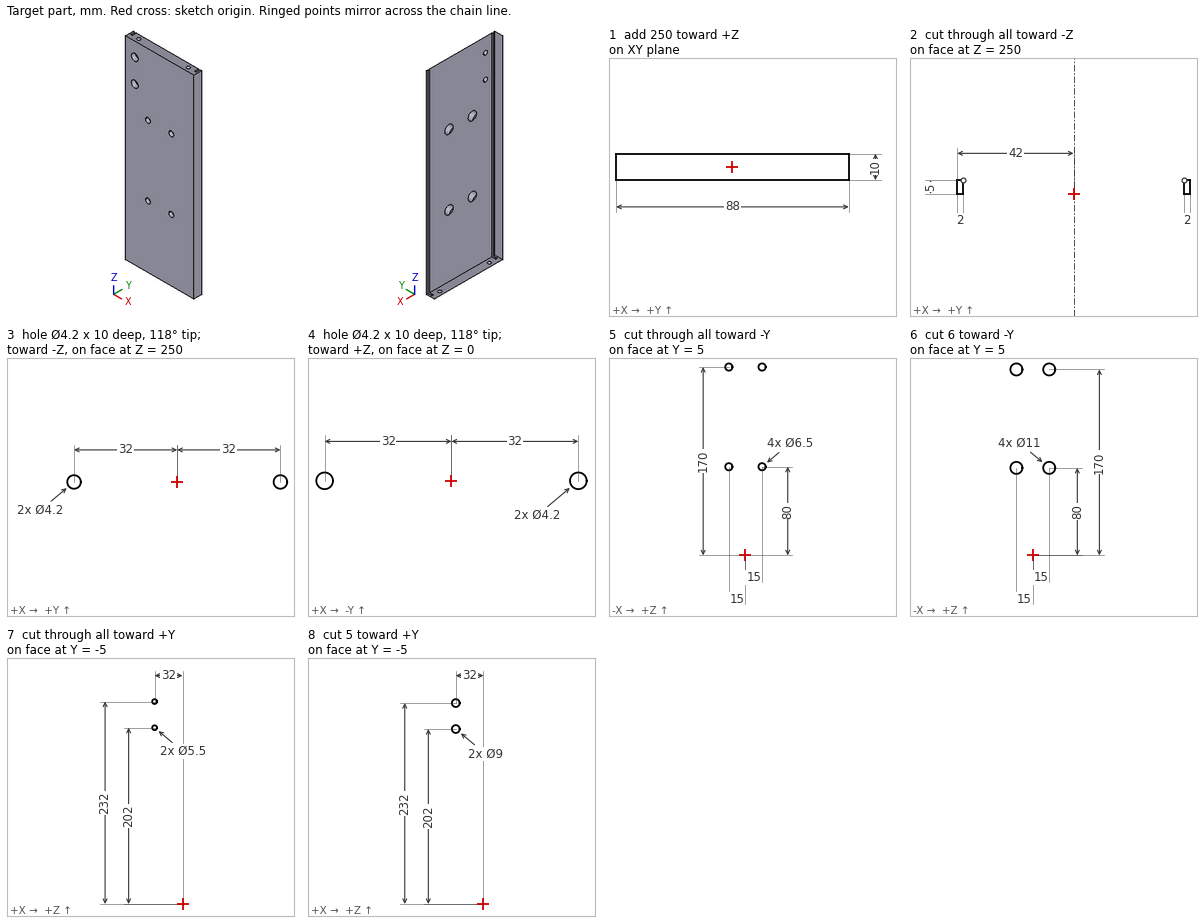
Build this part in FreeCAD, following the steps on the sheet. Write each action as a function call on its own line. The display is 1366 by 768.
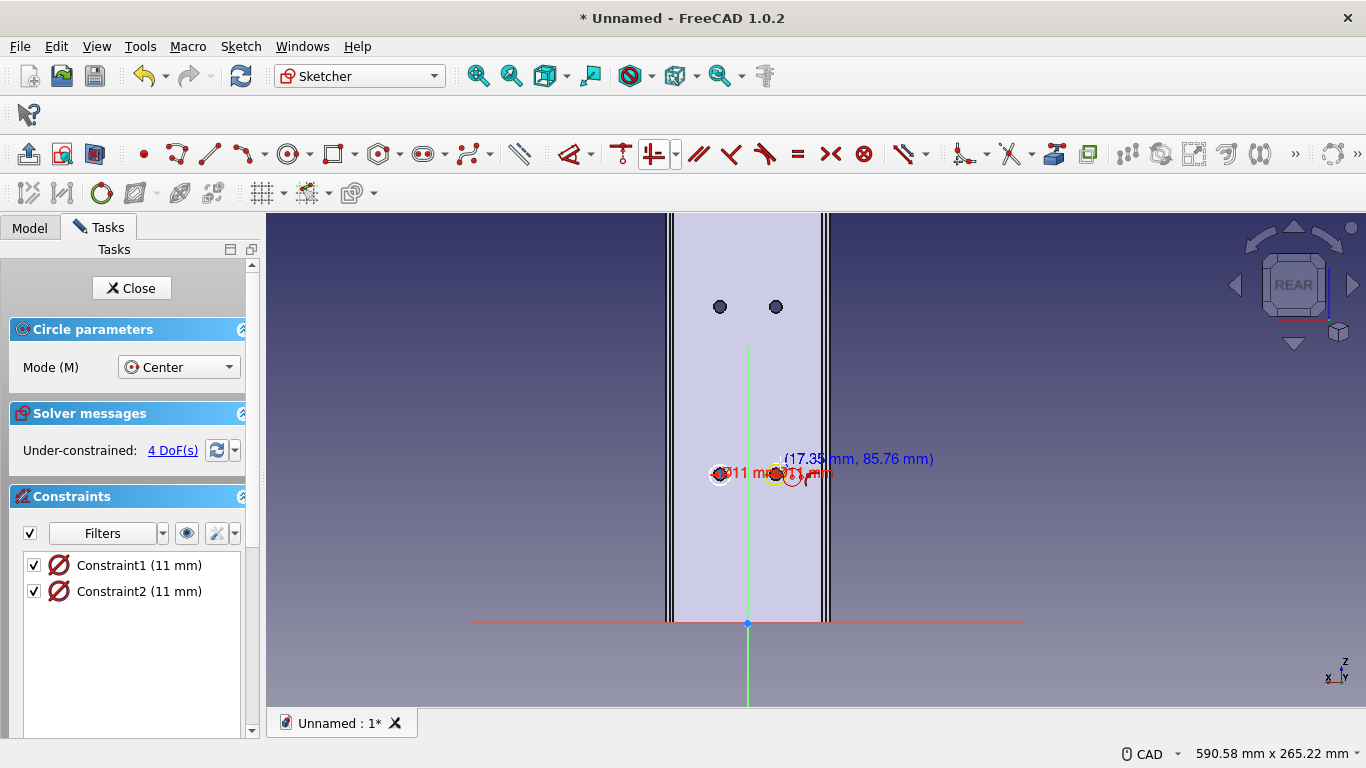
scroll(776, 307, up, 4)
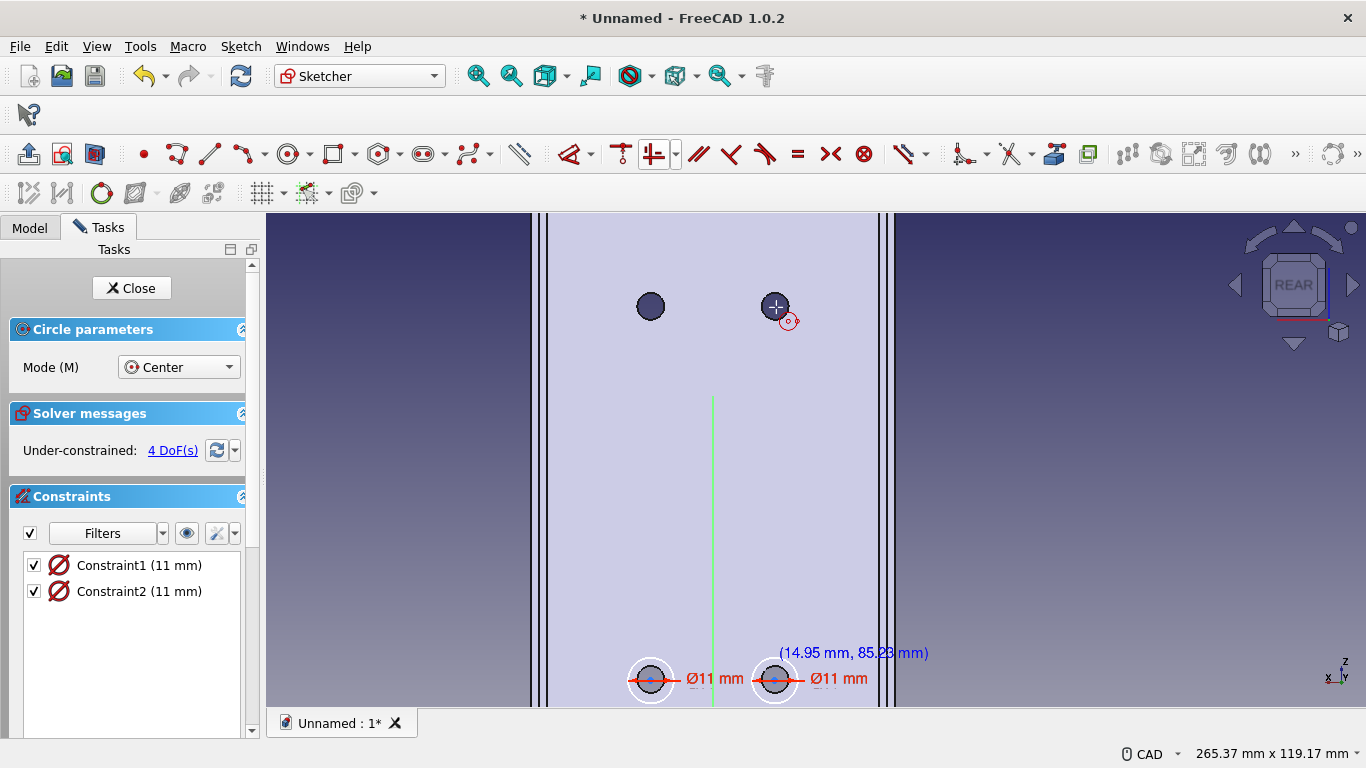
click(775, 306)
move(791, 290)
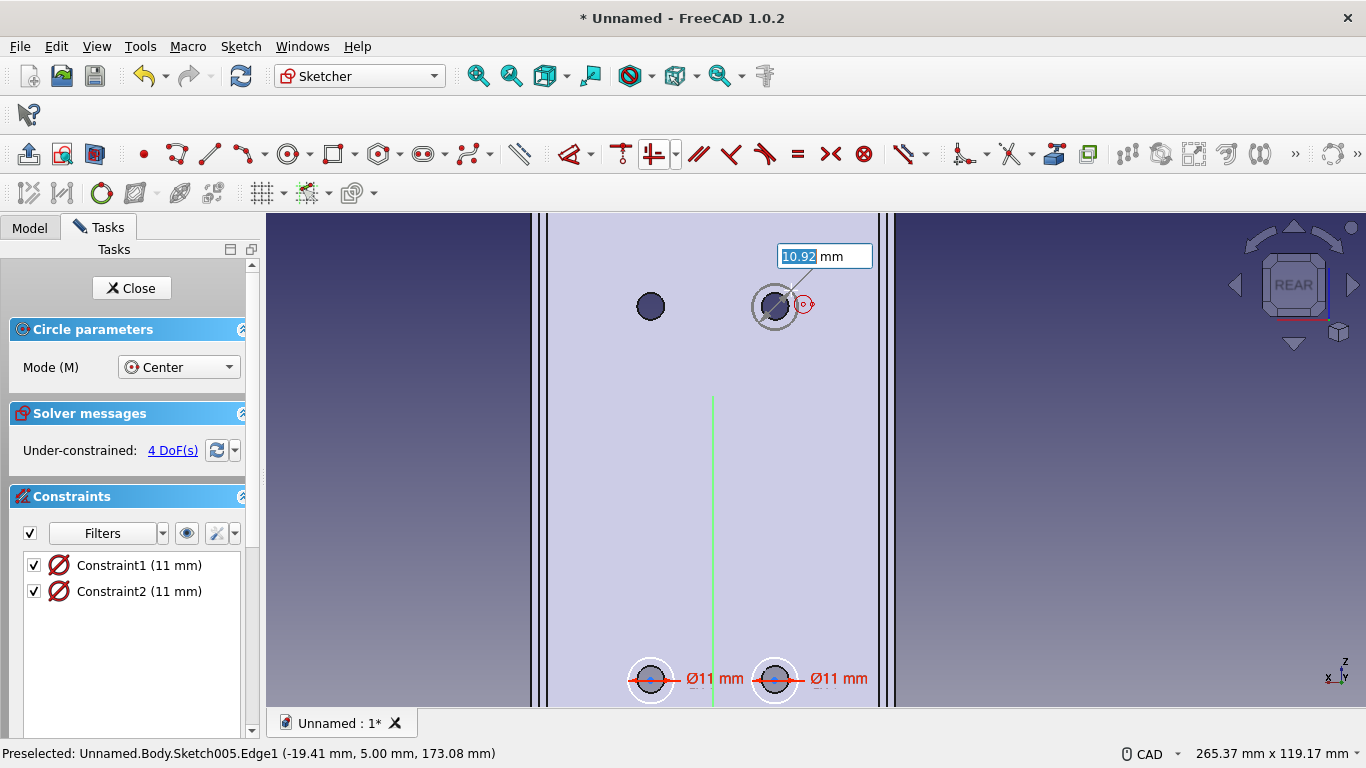
text(11)
key(Return)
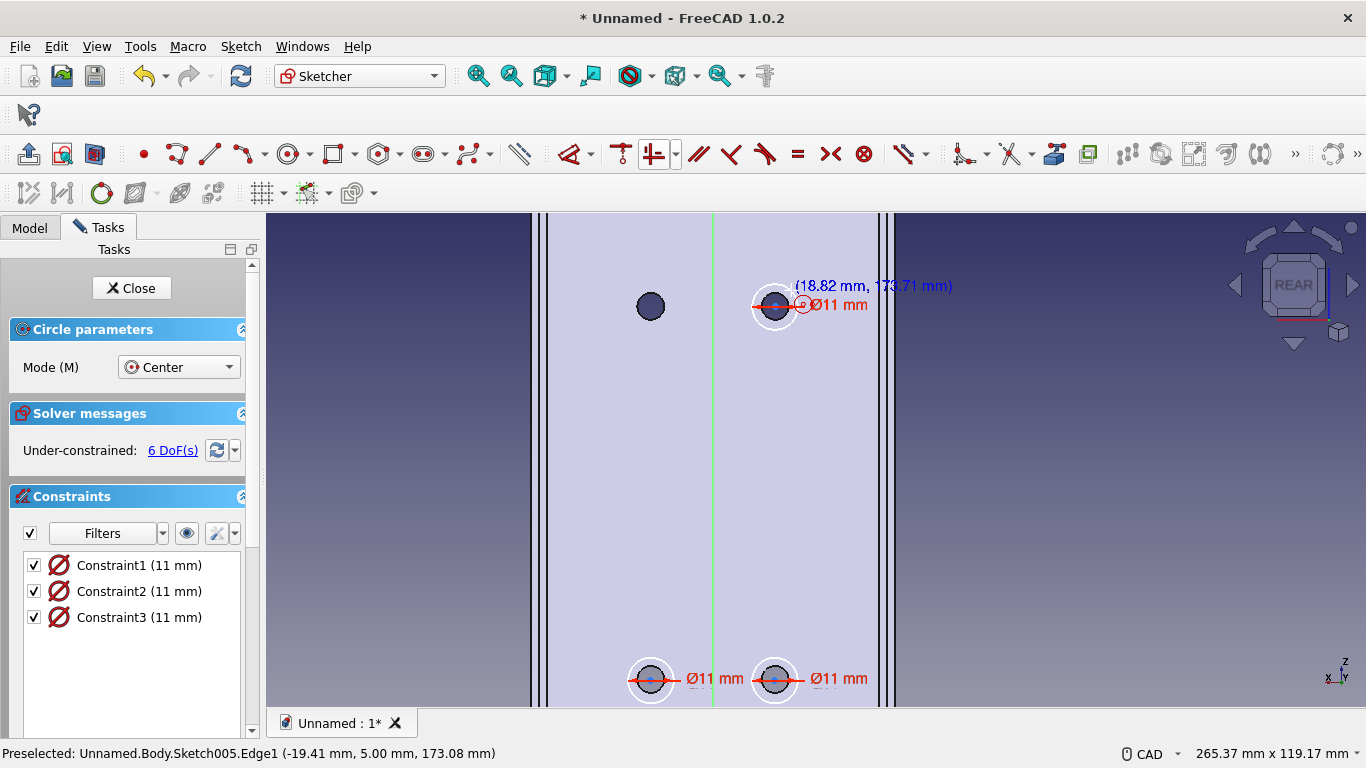
click(651, 306)
move(667, 290)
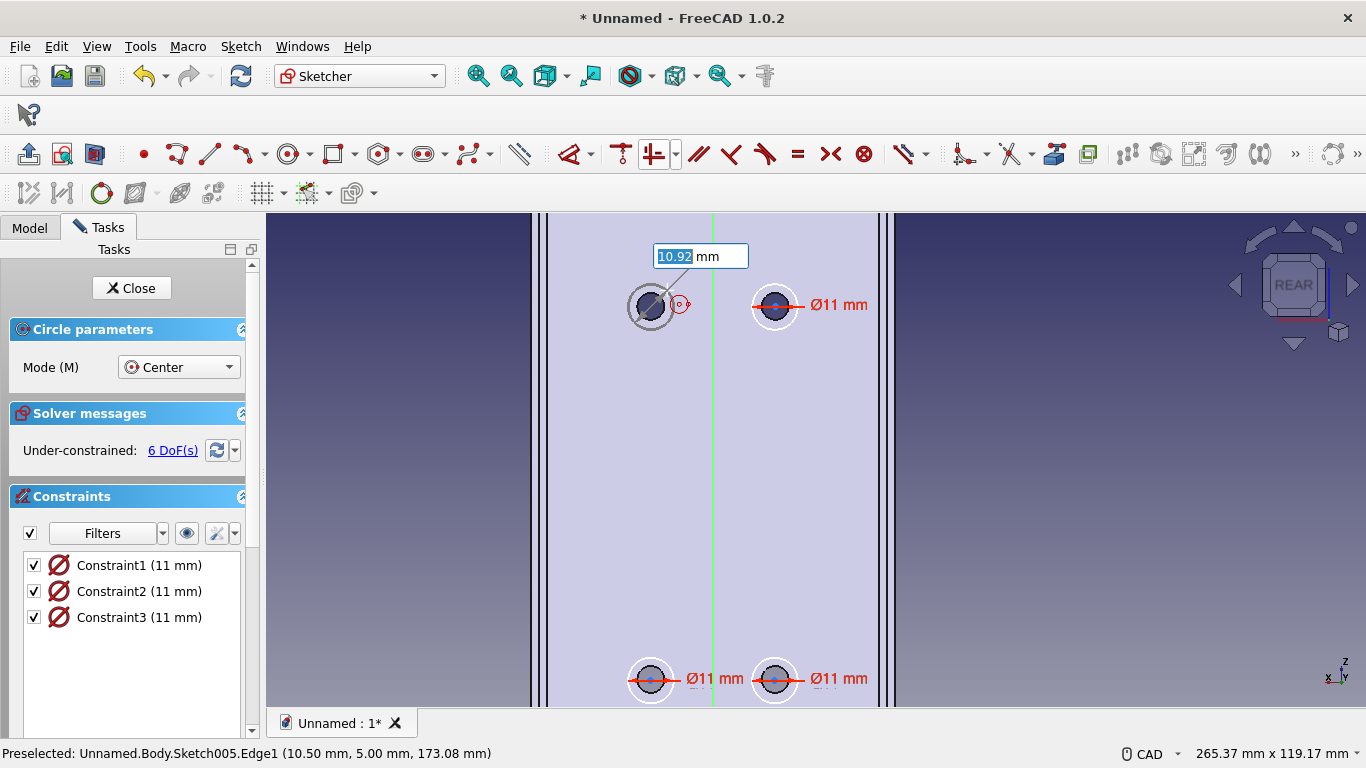
text(11)
key(Return)
key(Escape)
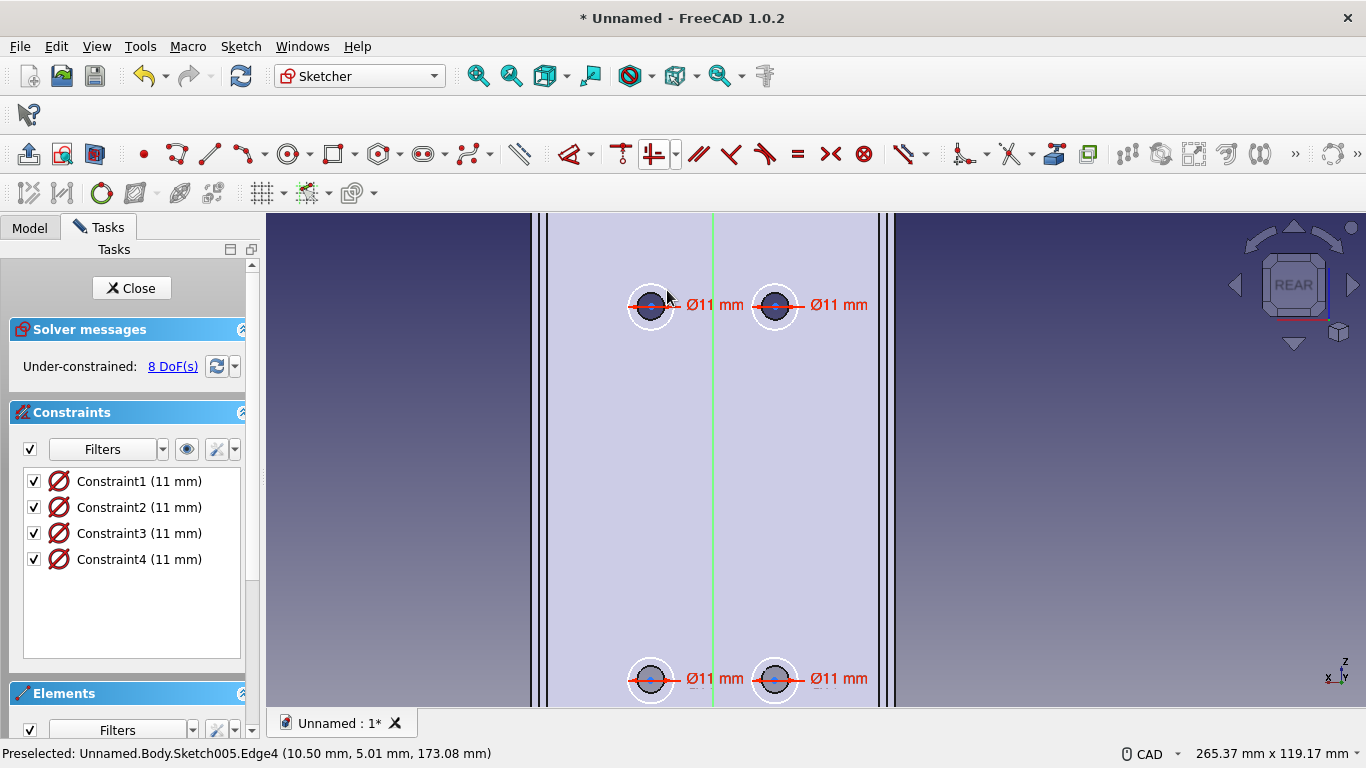
scroll(776, 307, down, 4)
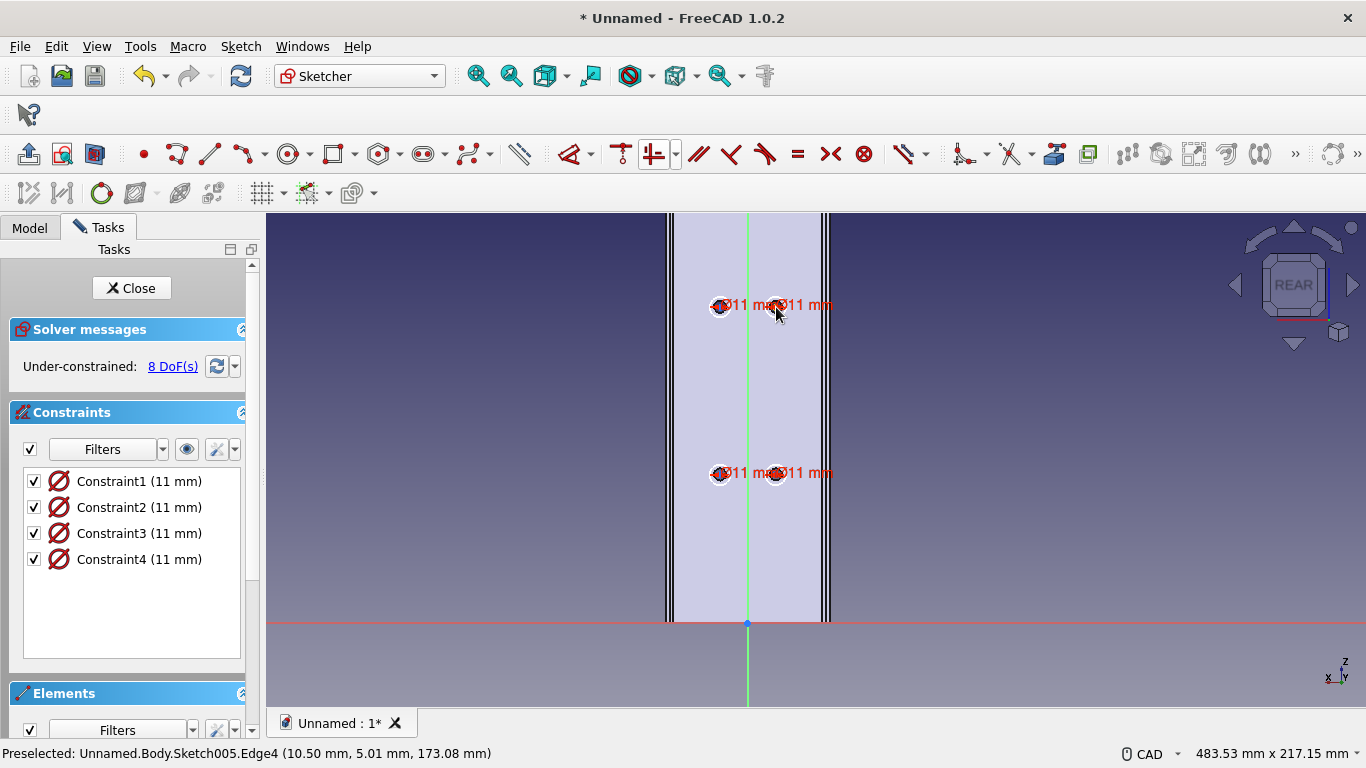
click(776, 475)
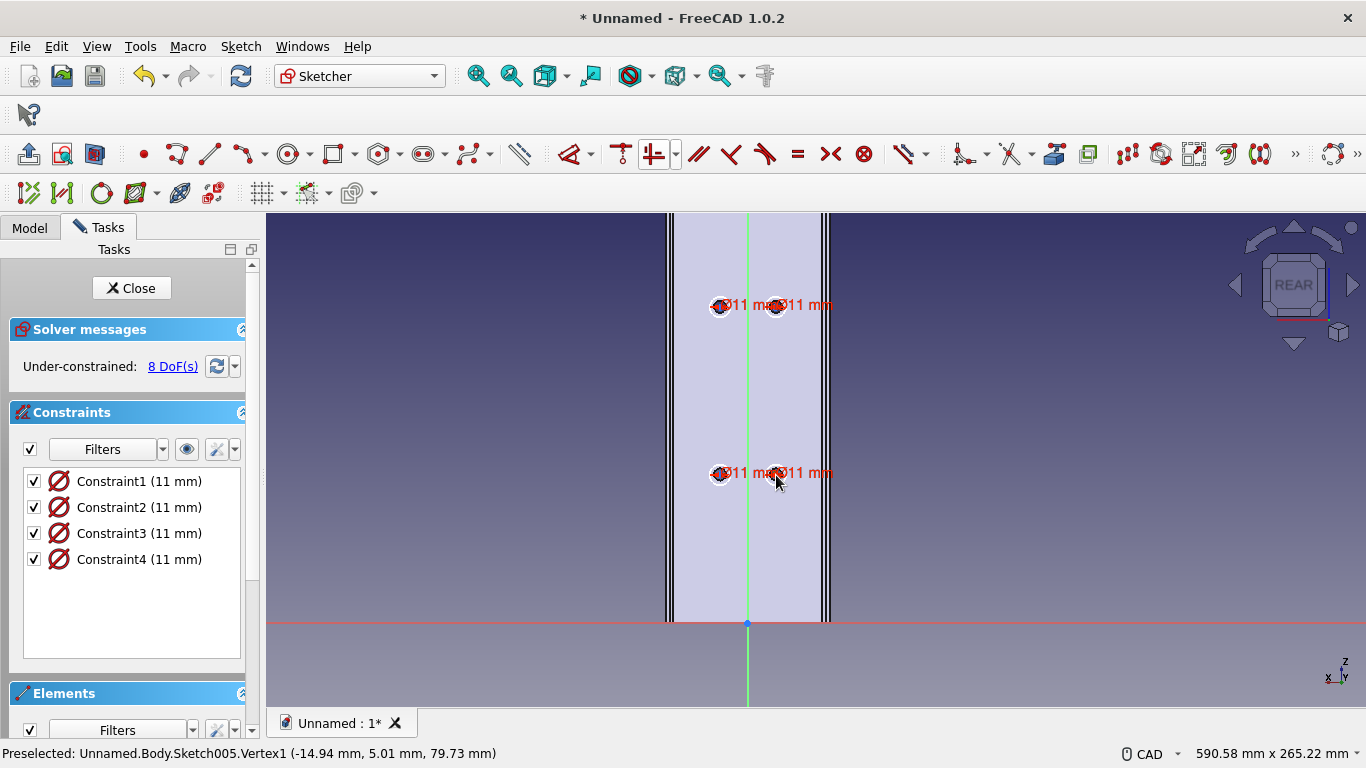
click(720, 475)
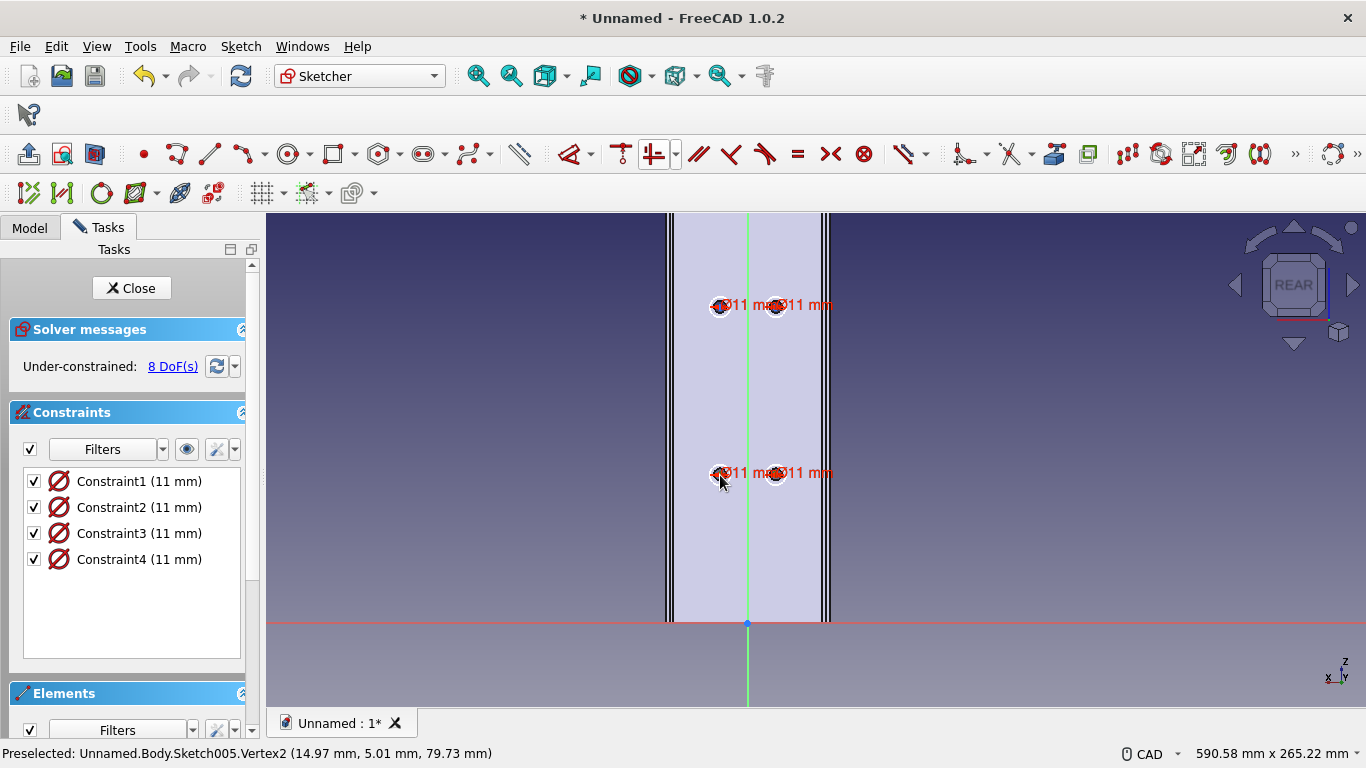
click(676, 154)